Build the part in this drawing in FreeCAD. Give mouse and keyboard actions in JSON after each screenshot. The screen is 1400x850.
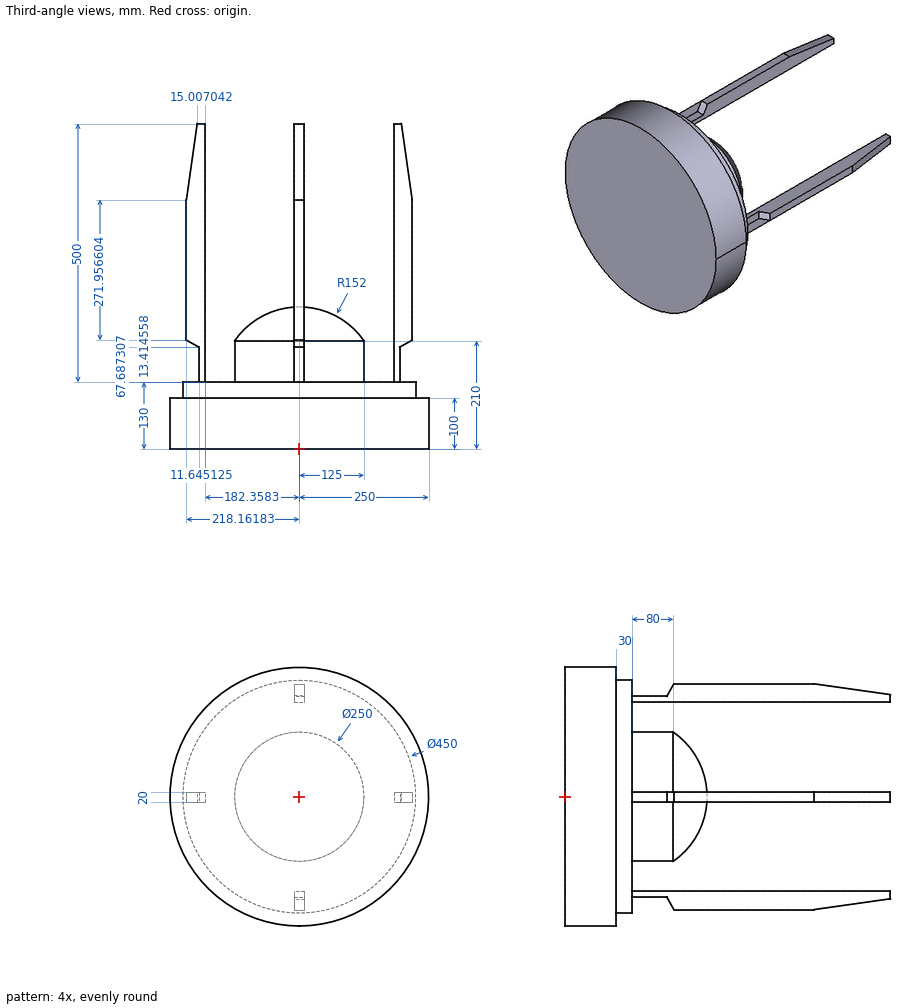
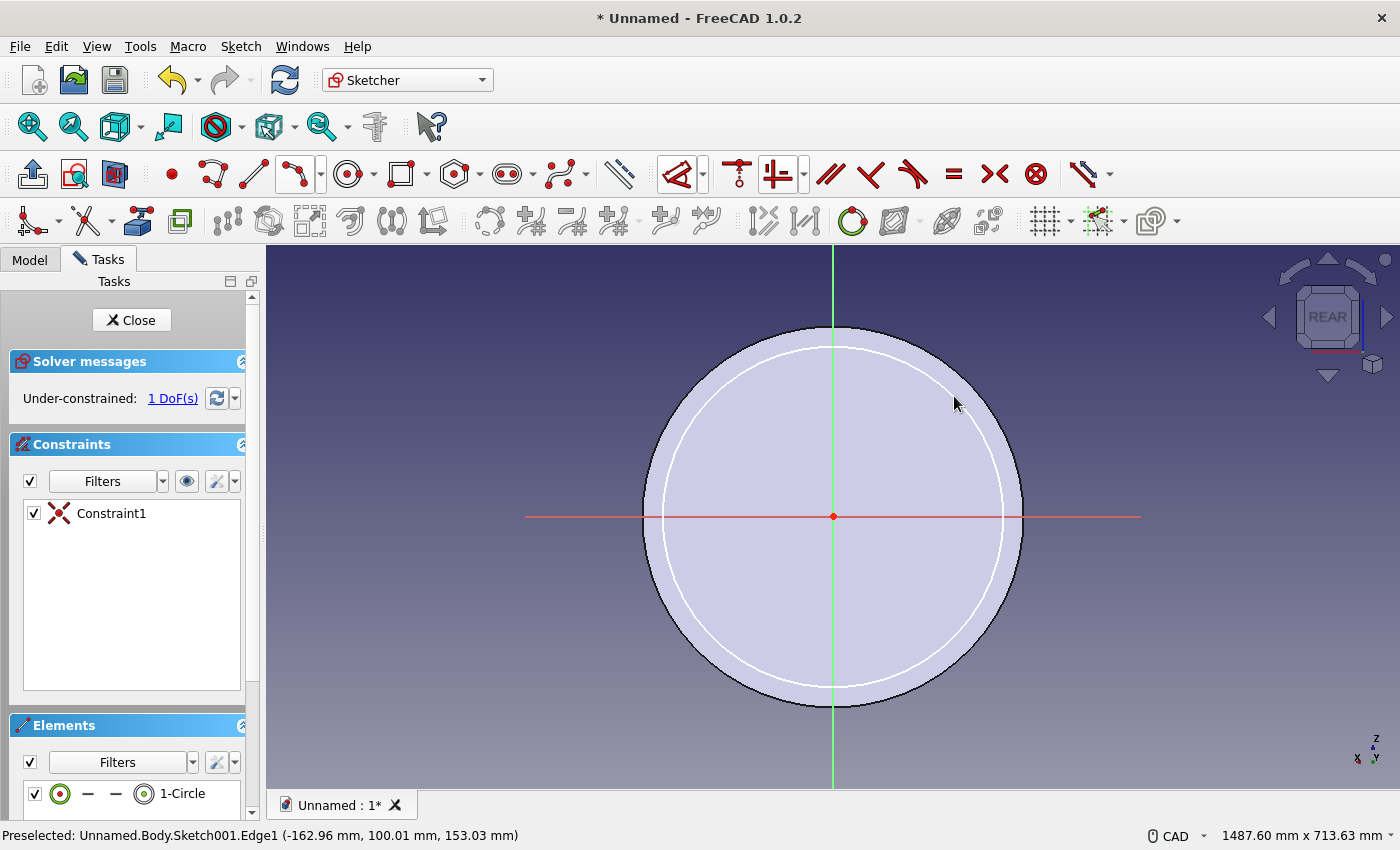
{"action": "left_click", "coordinate": [953, 396]}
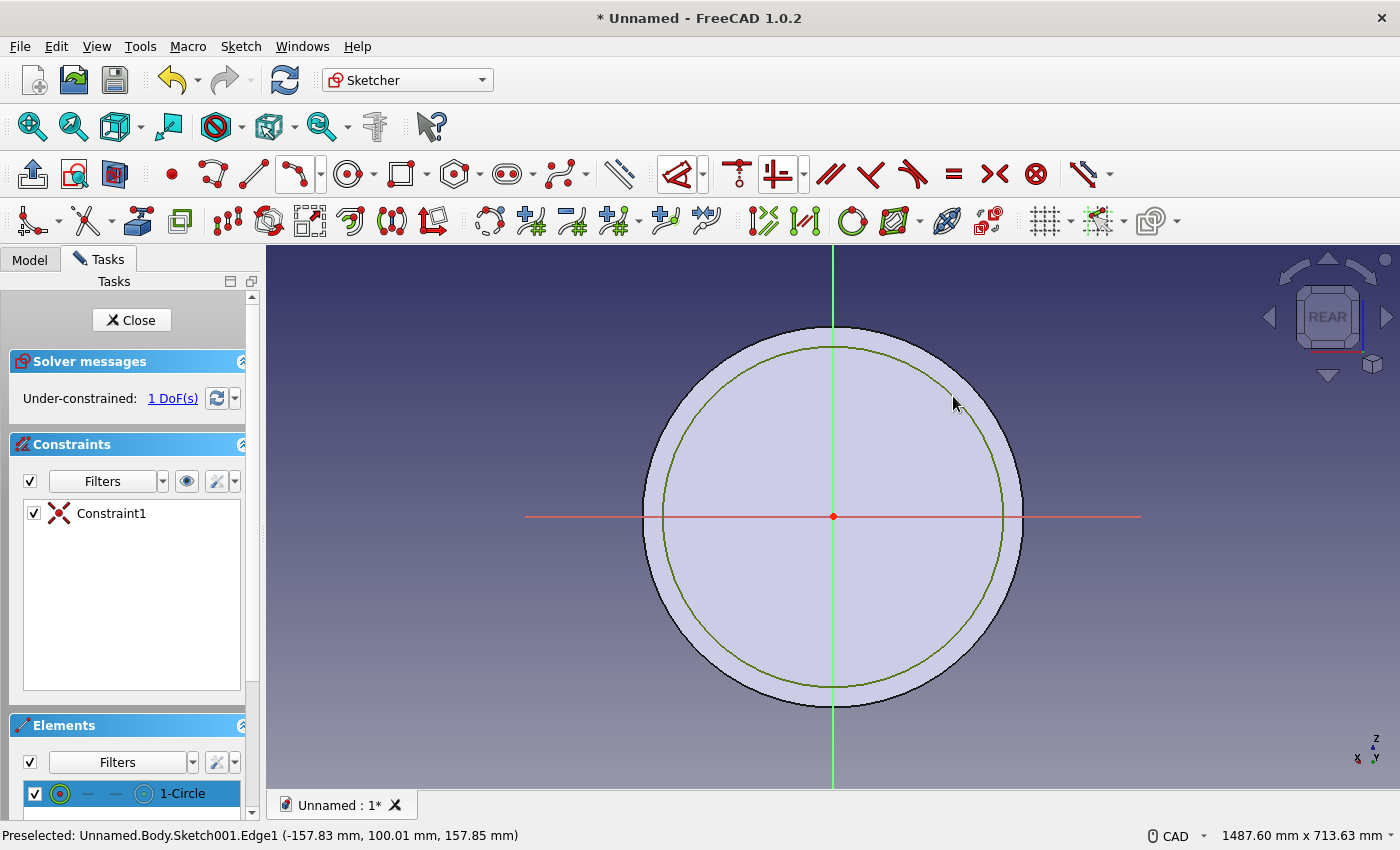
{"action": "key", "text": "k o"}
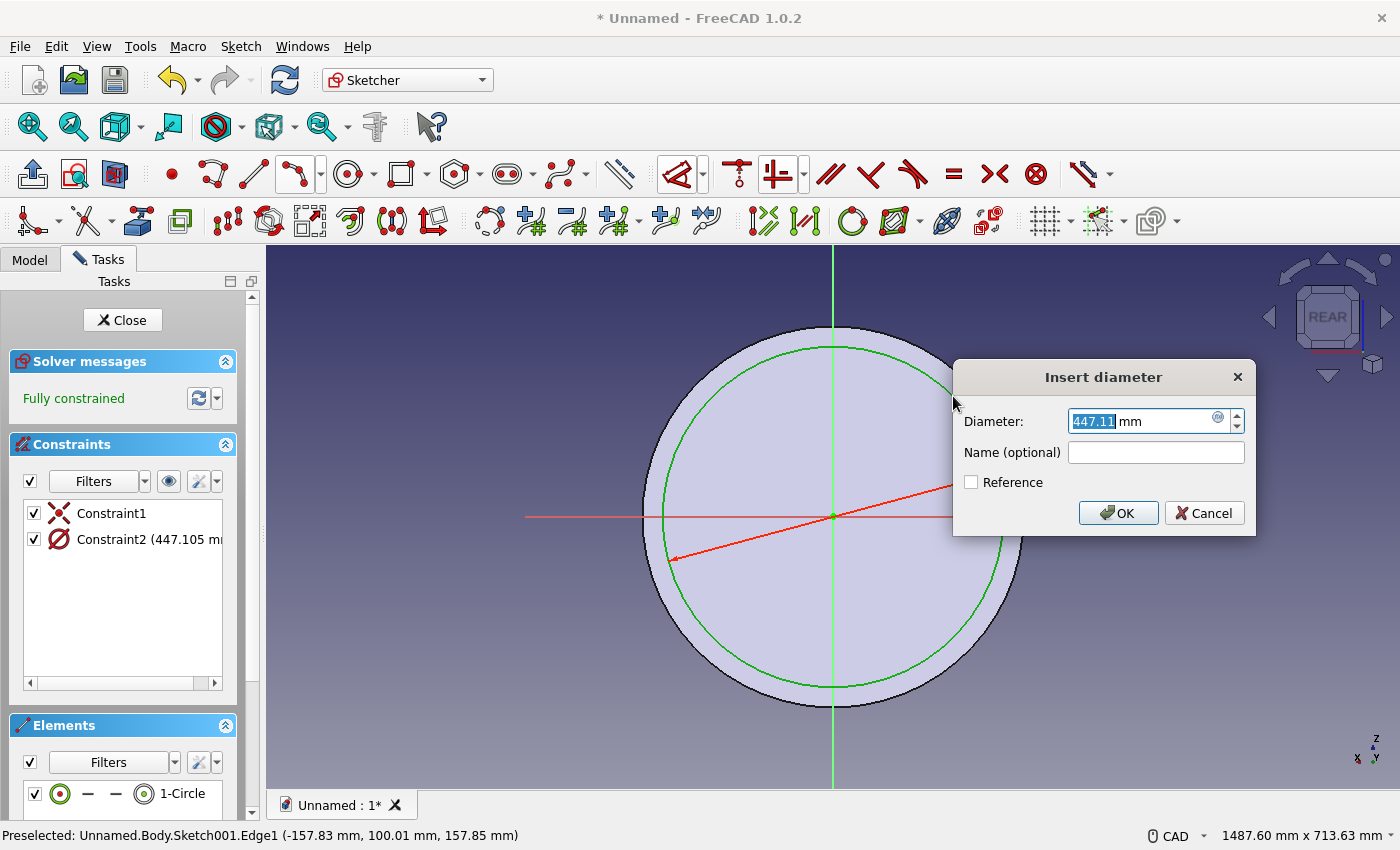
{"action": "type", "text": "450"}
{"action": "key", "text": "Return"}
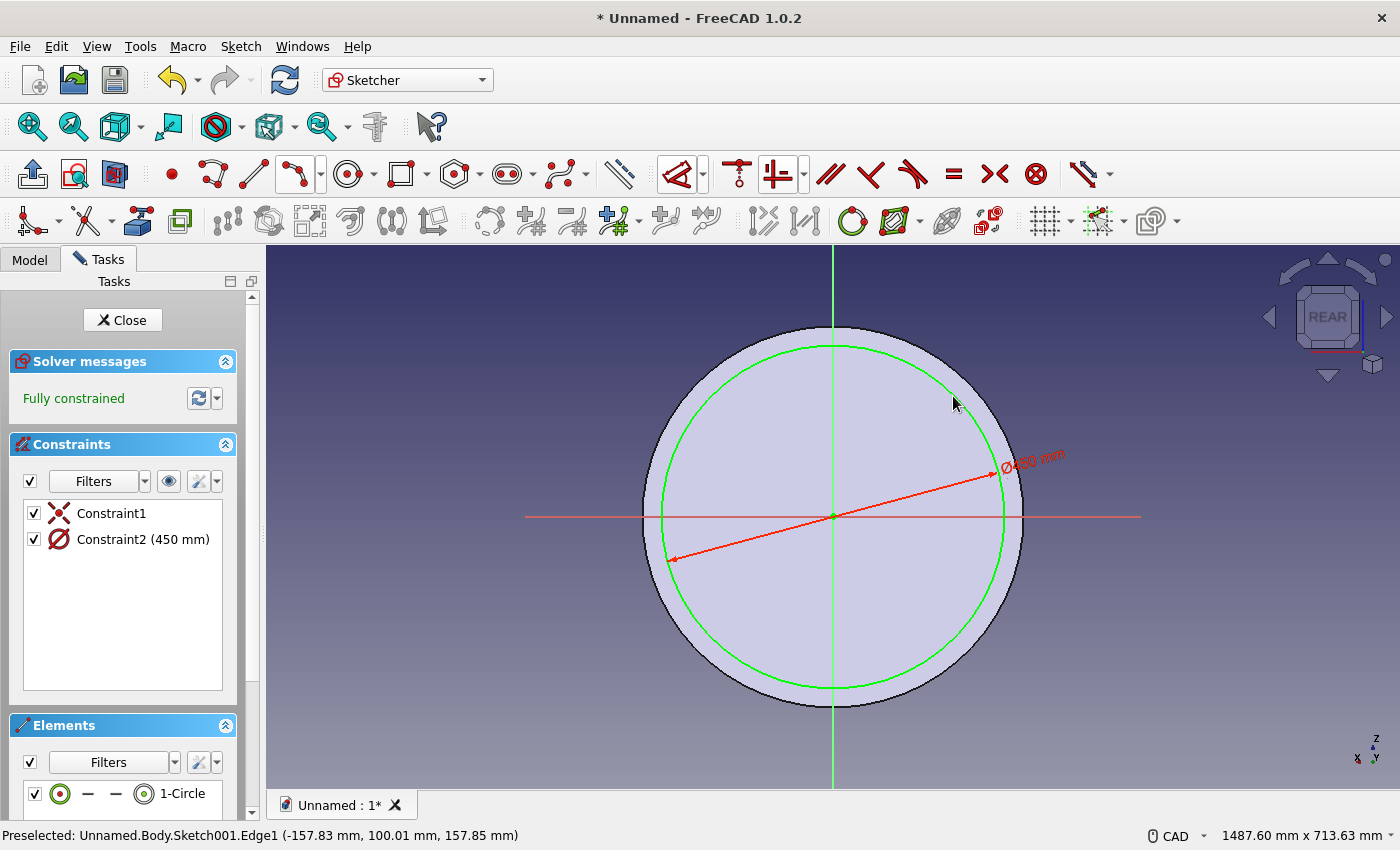
{"action": "left_click", "coordinate": [123, 320]}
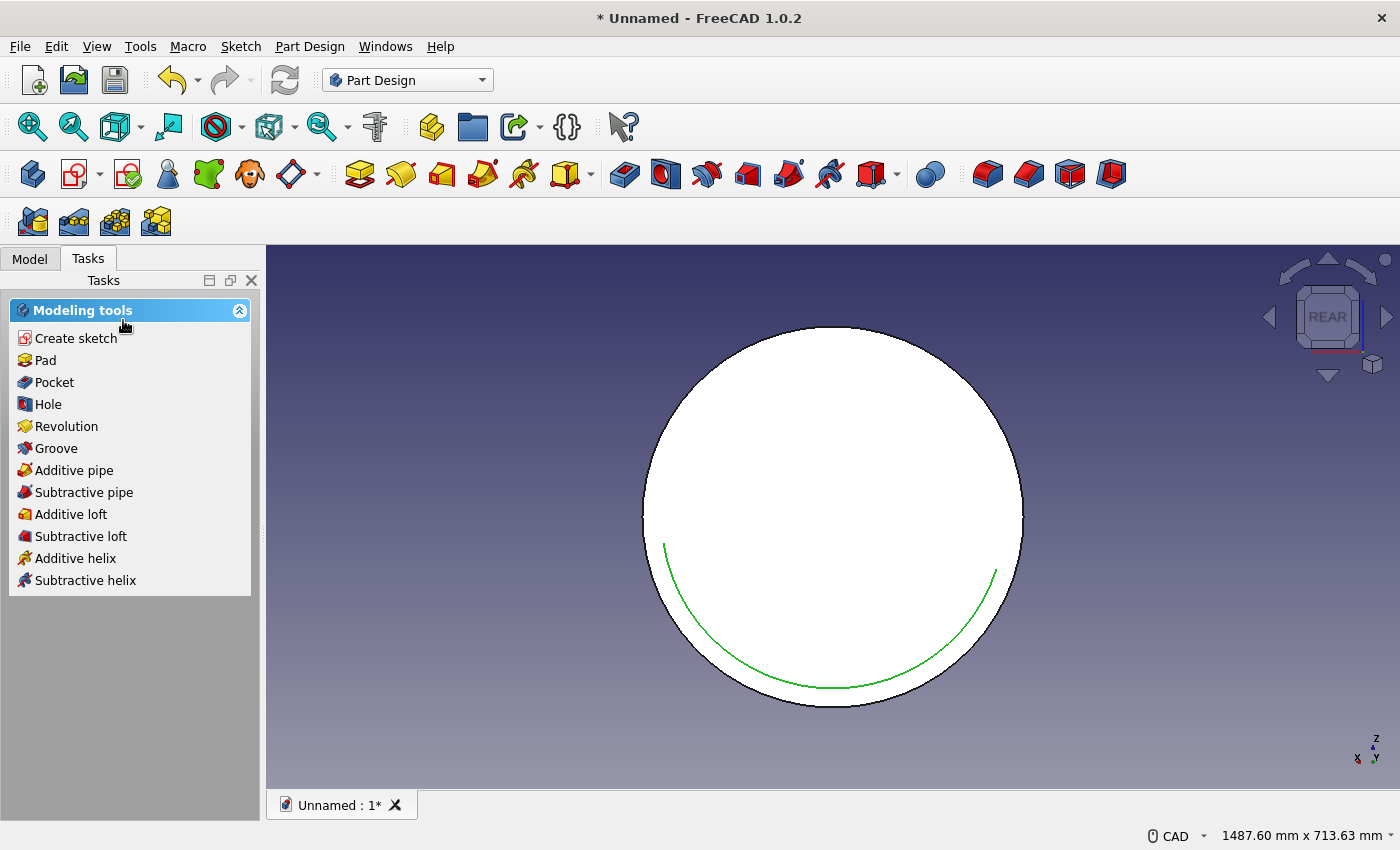
{"action": "left_click", "coordinate": [360, 174]}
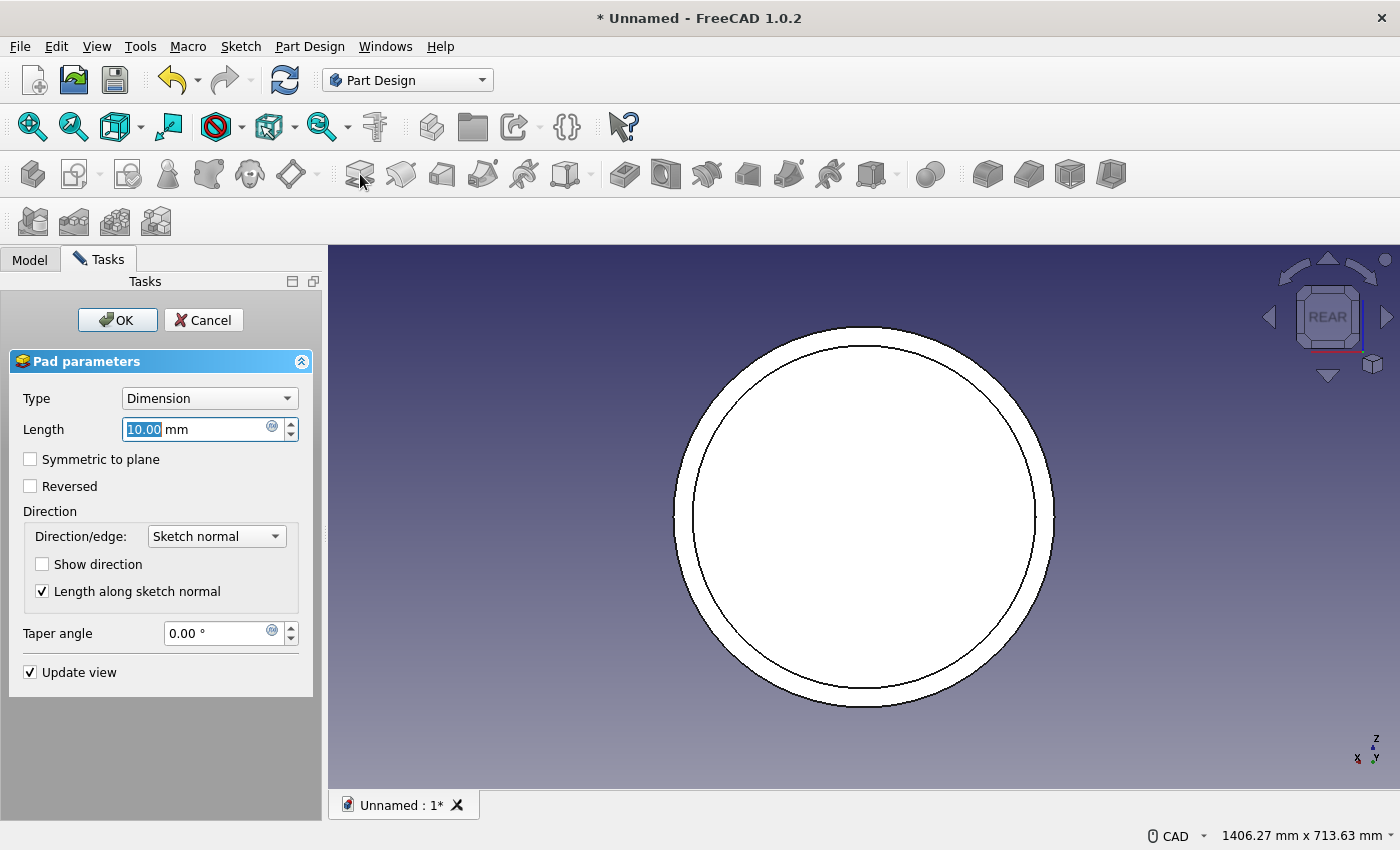
{"action": "type", "text": "30"}
{"action": "key", "text": "Tab"}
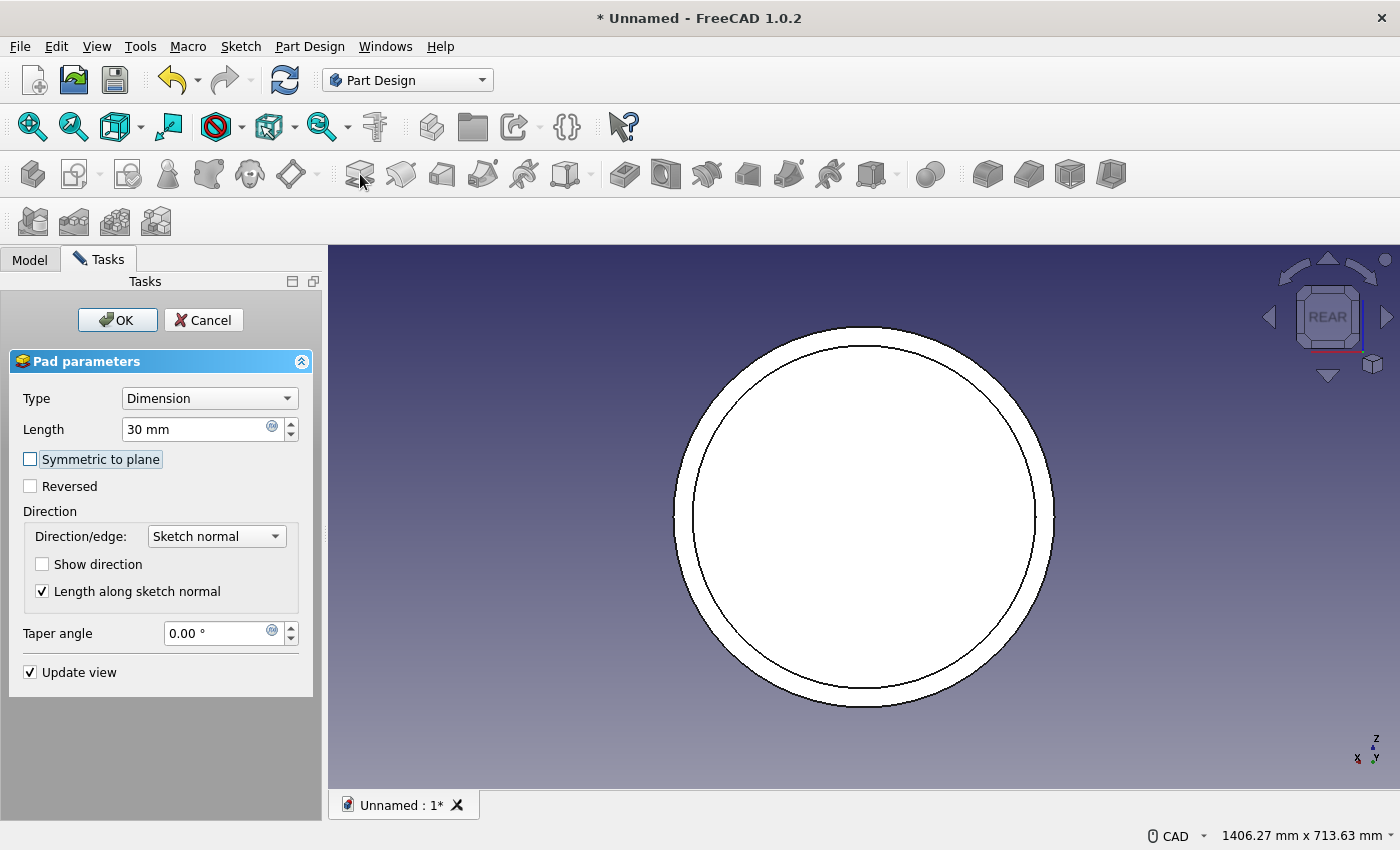
{"action": "left_click", "coordinate": [118, 320]}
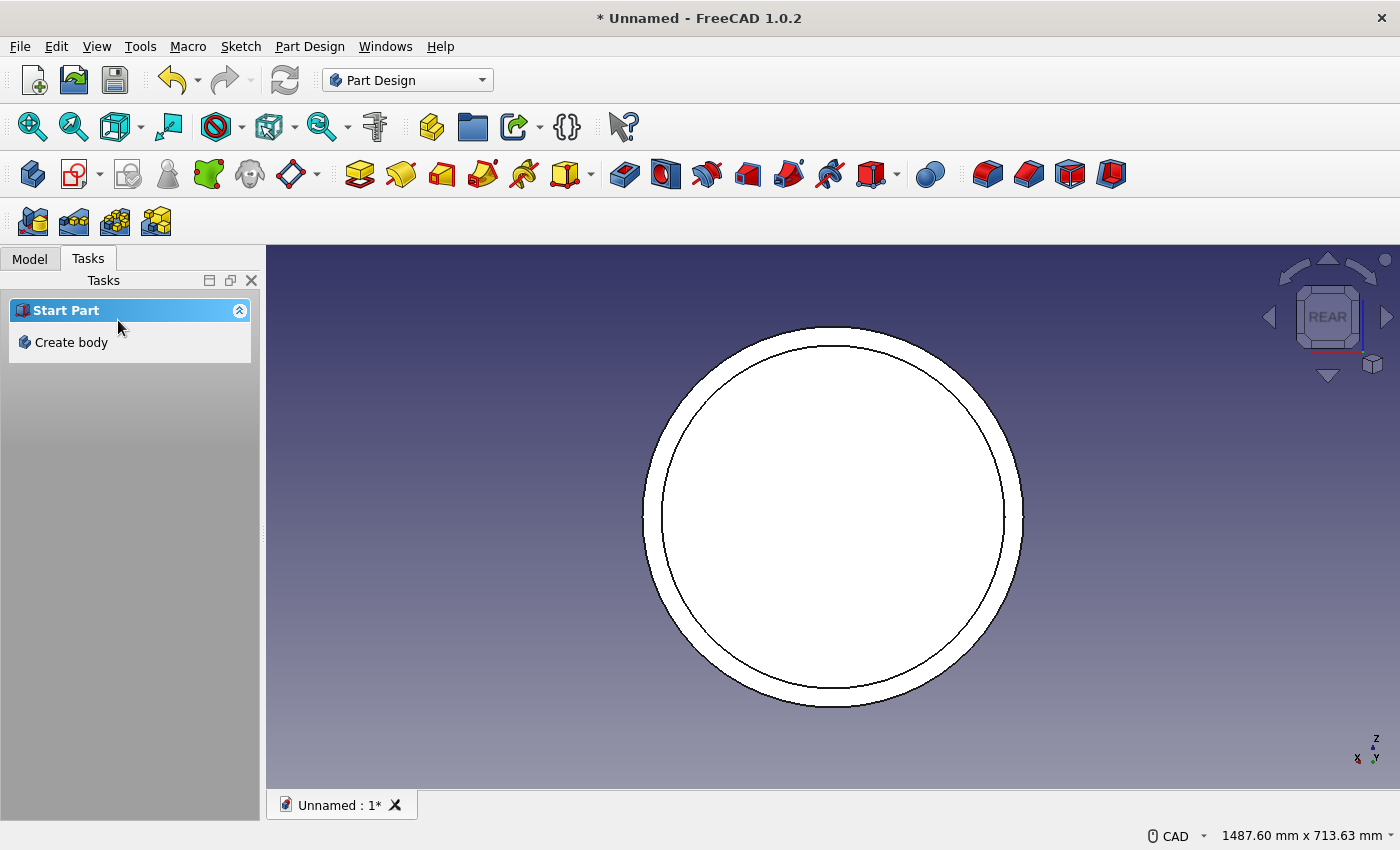
{"action": "left_click", "coordinate": [833, 516]}